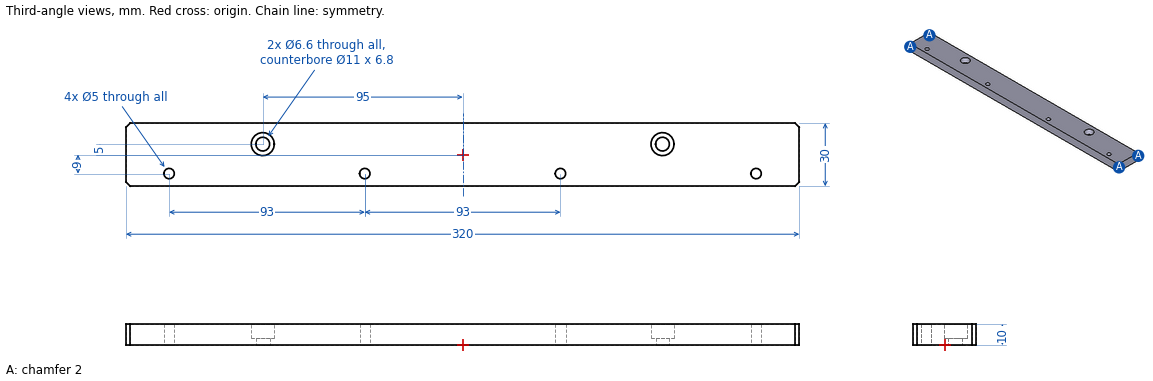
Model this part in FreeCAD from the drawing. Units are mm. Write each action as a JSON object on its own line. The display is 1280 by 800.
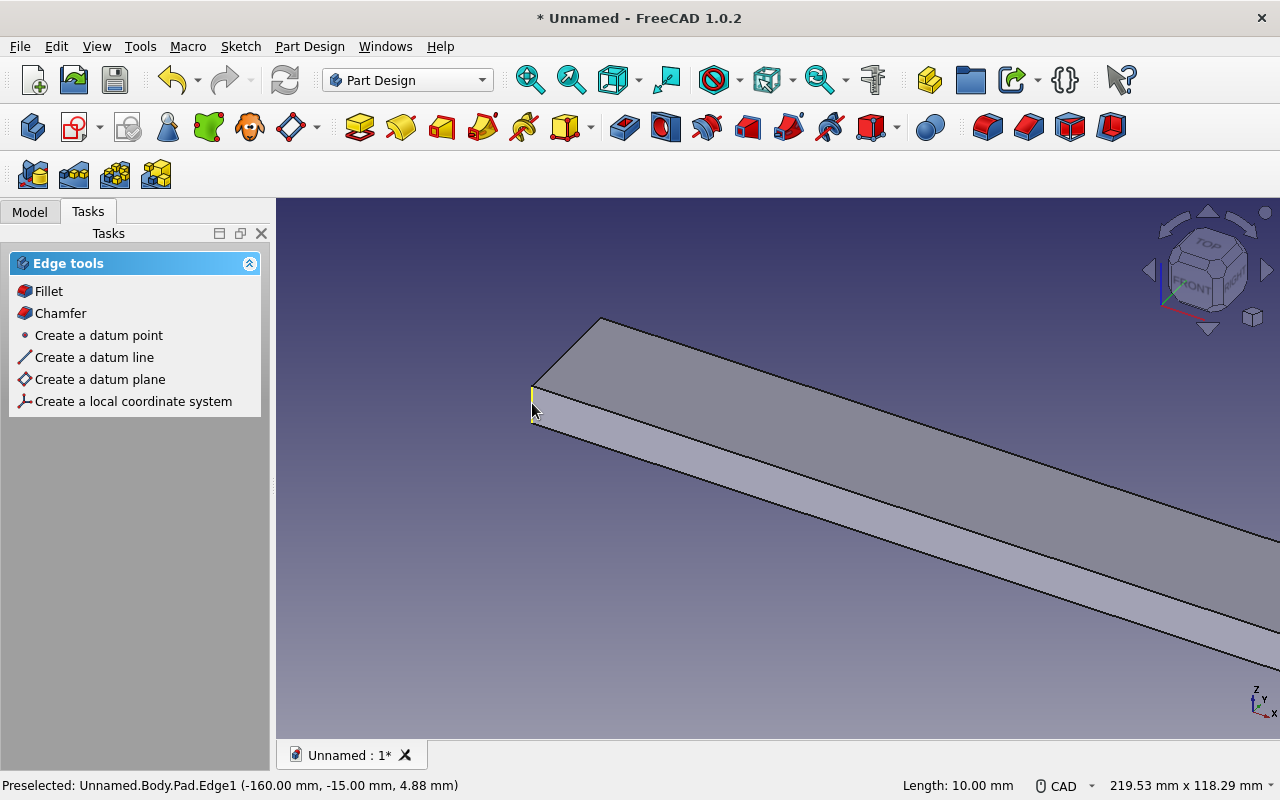
{"action": "left_click", "coordinate": [531, 80]}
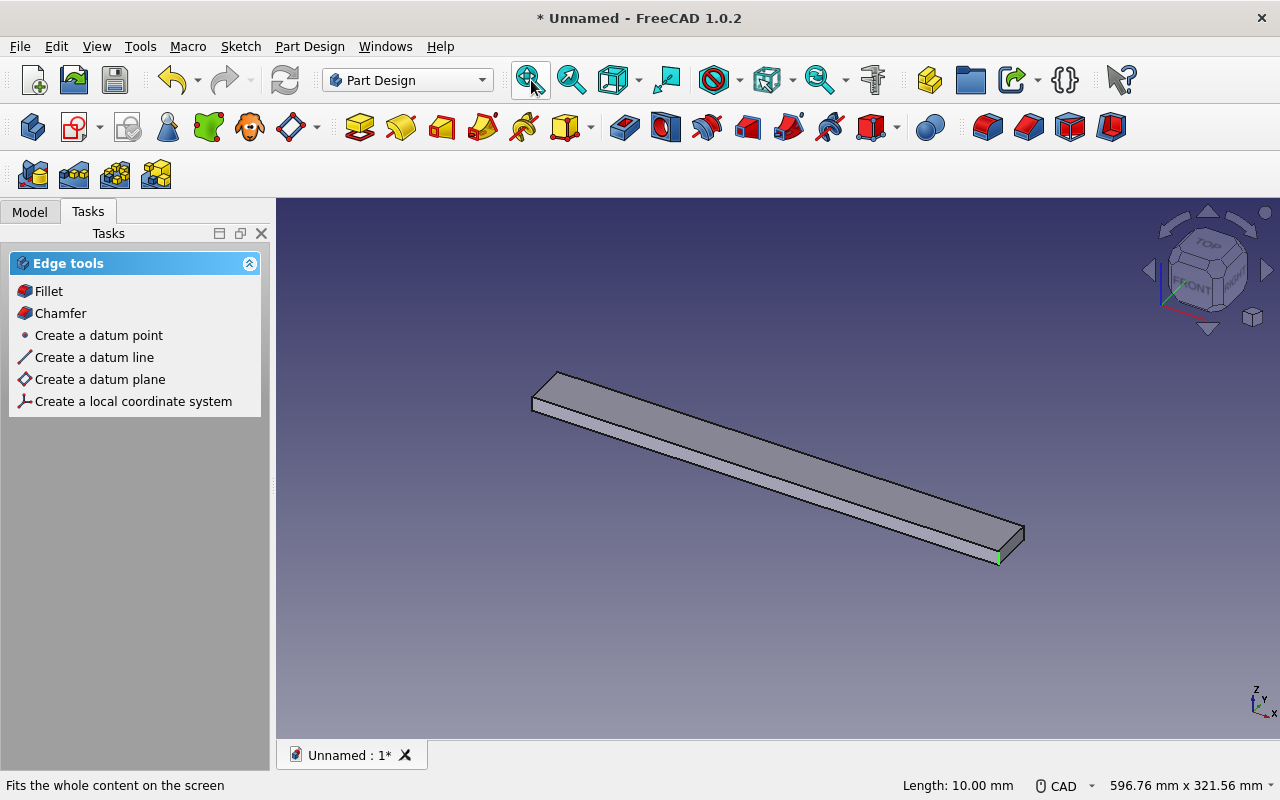
{"action": "key", "text": "0"}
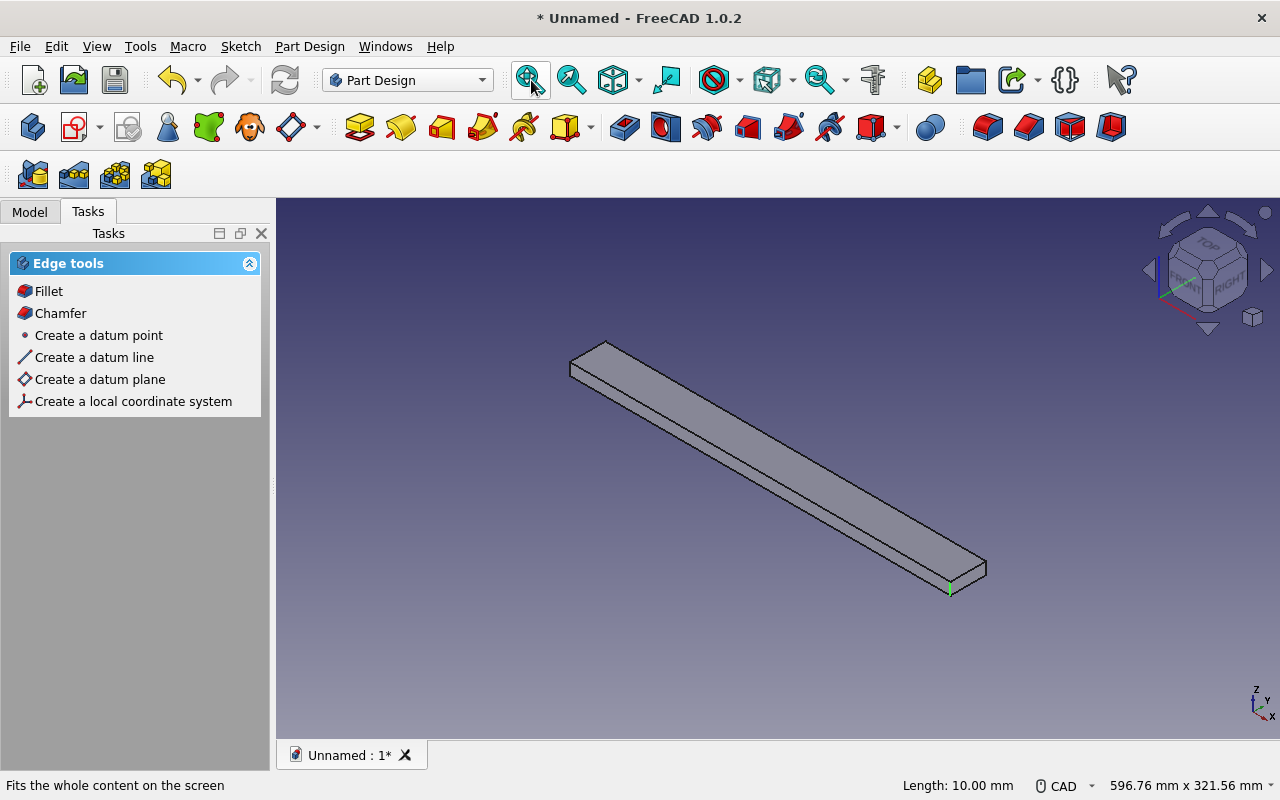
{"action": "scroll", "coordinate": [570, 368], "scroll_direction": "up", "scroll_amount": 5}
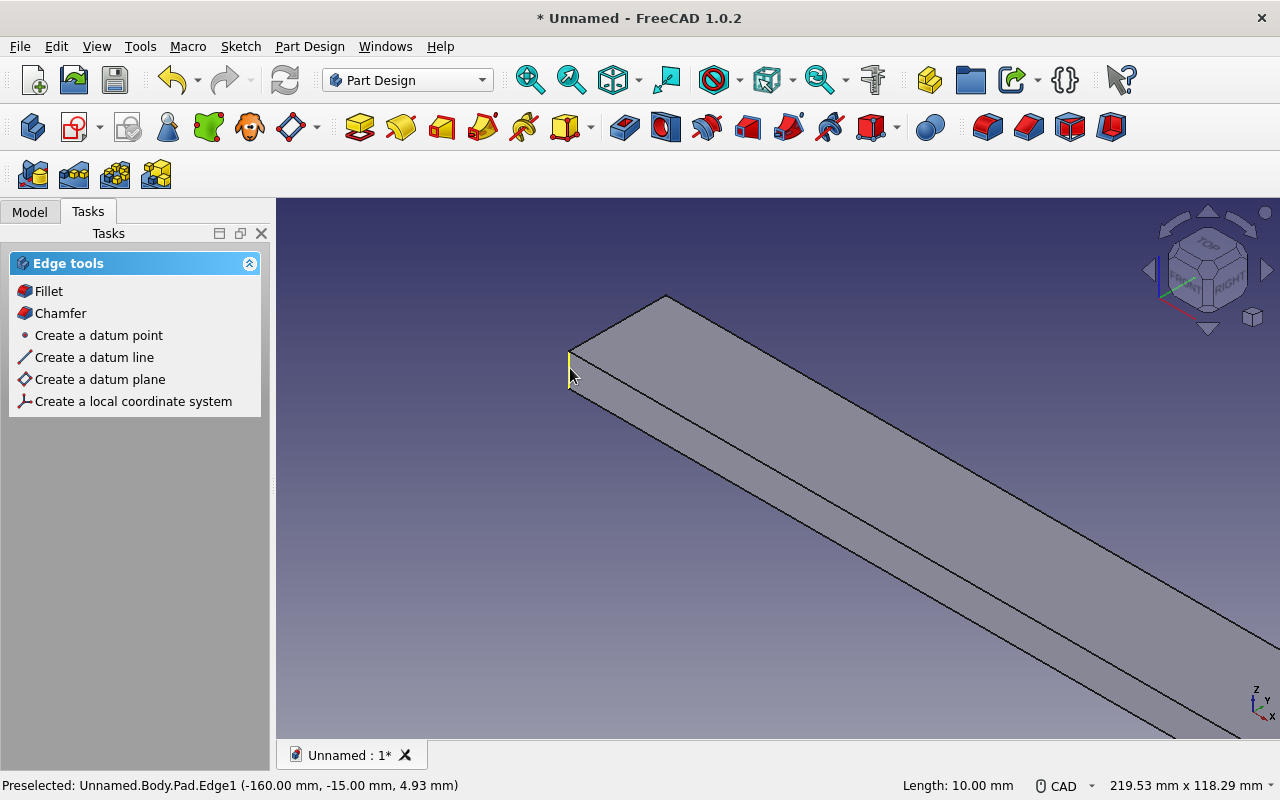
{"action": "left_click", "coordinate": [531, 80]}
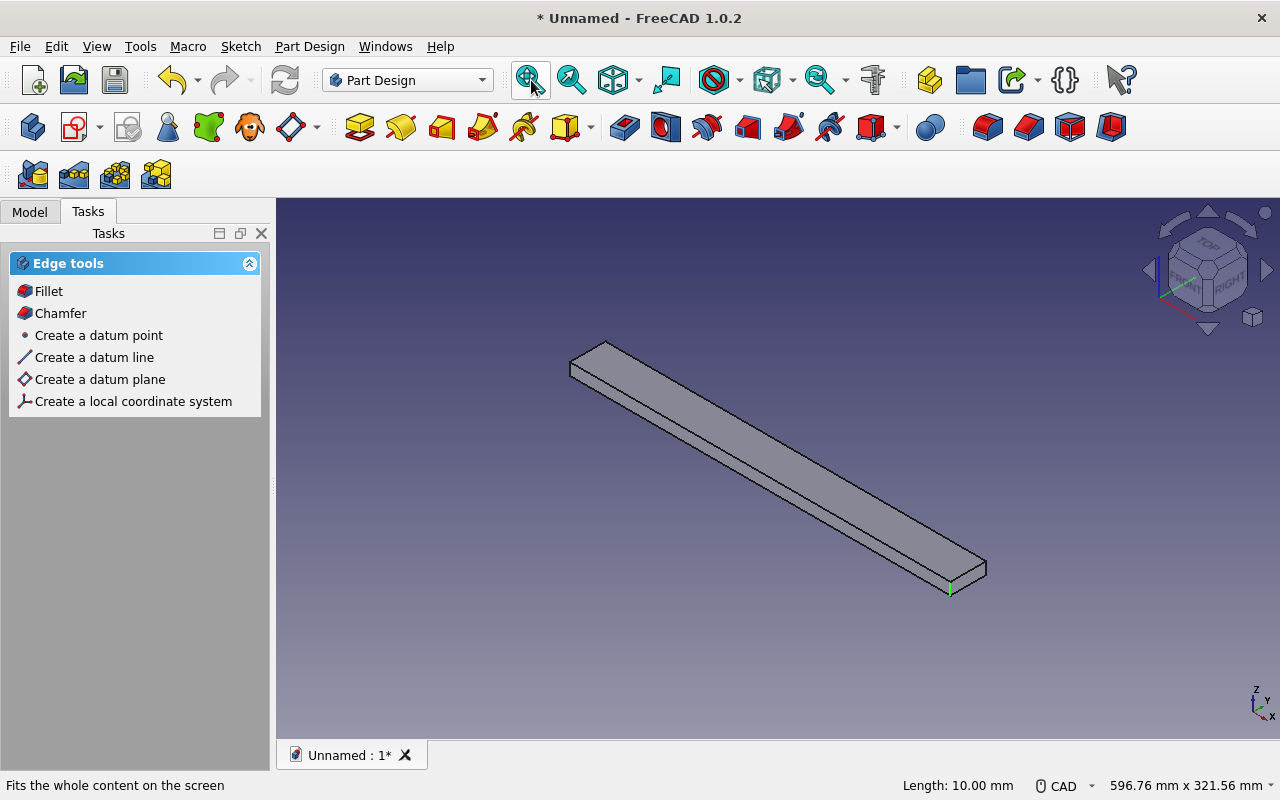
{"action": "key", "text": "2"}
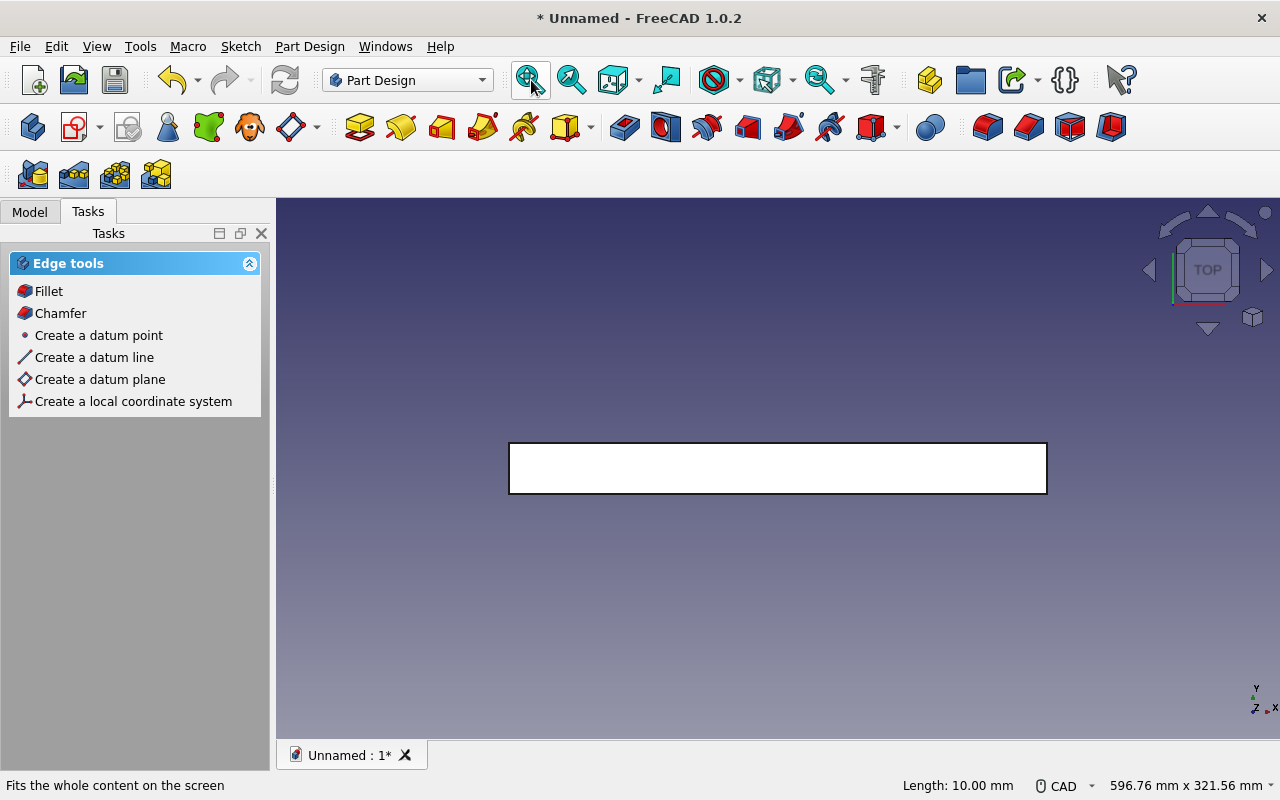
{"action": "scroll", "coordinate": [509, 493], "scroll_direction": "up", "scroll_amount": 5}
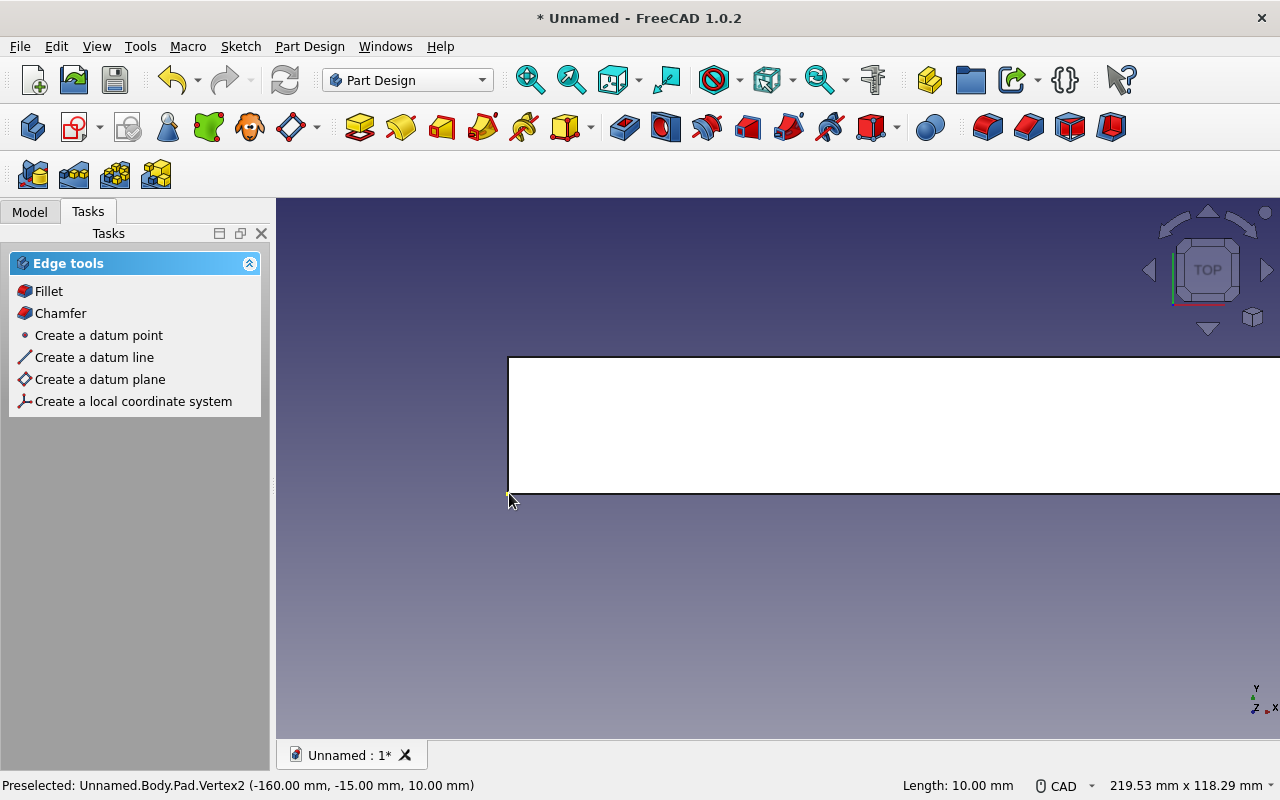
{"action": "left_click", "coordinate": [531, 80]}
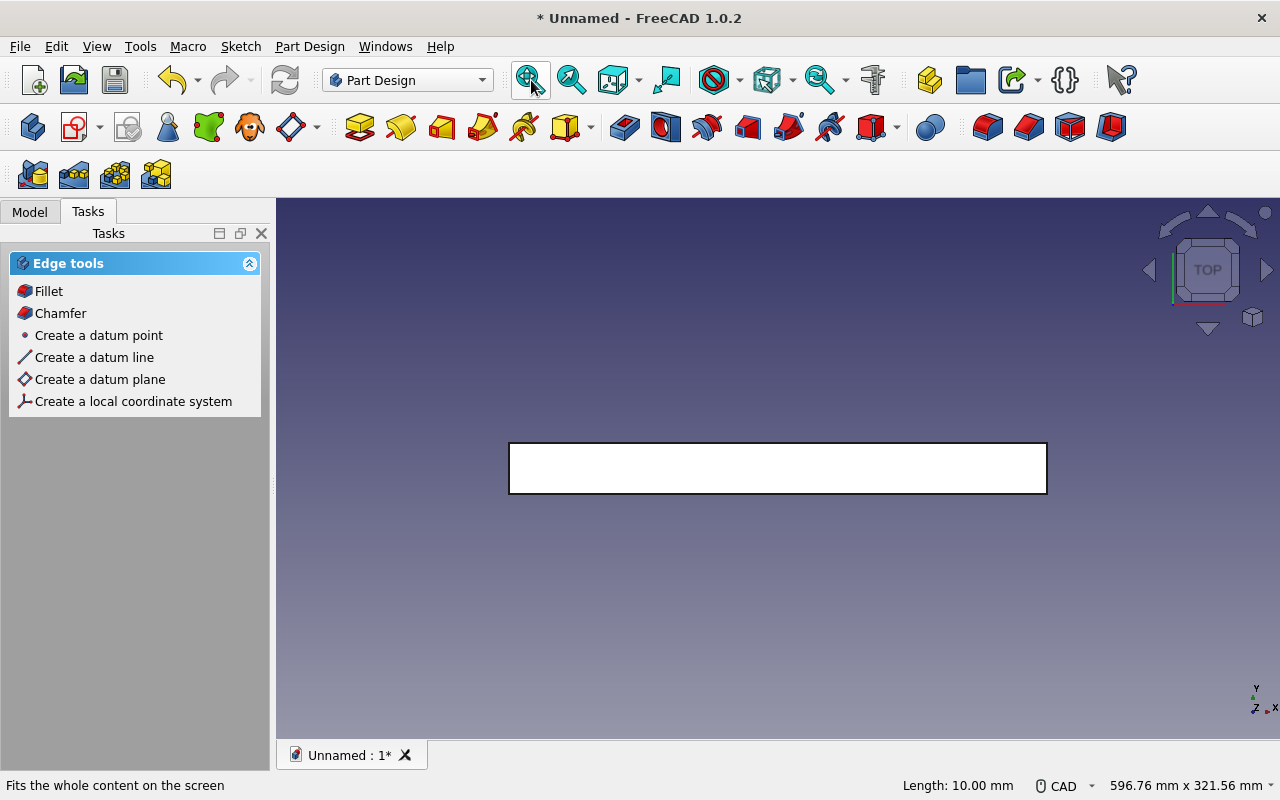
{"action": "key", "text": "1"}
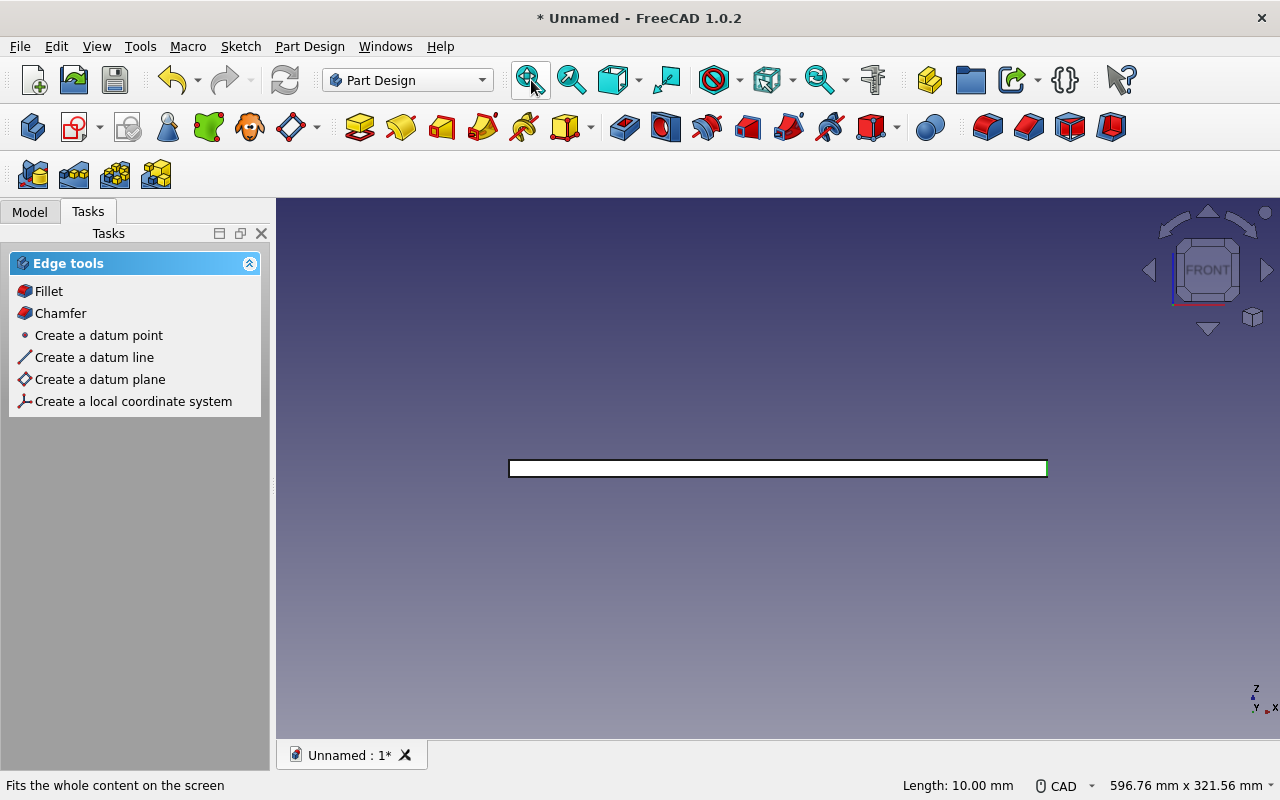
{"action": "left_click", "coordinate": [509, 467], "text": "ctrl"}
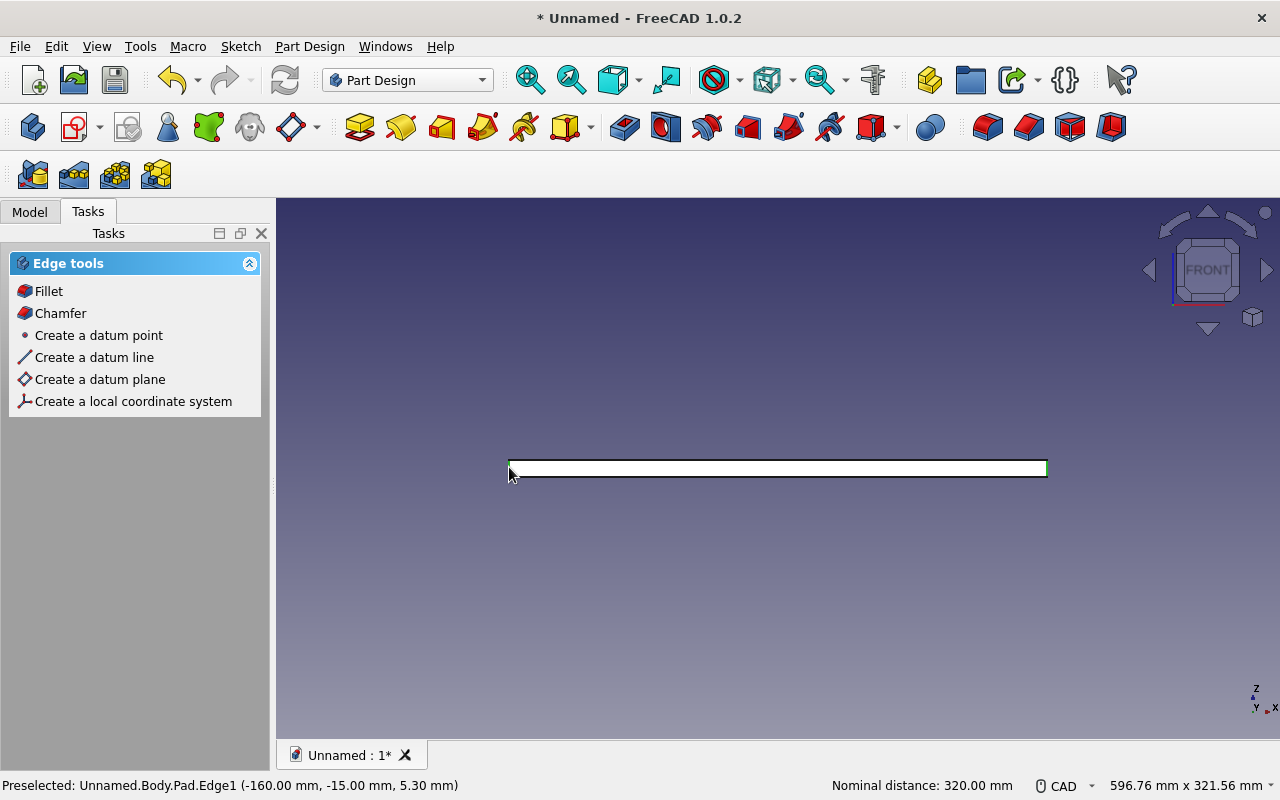
{"action": "scroll", "coordinate": [509, 467], "scroll_direction": "up", "scroll_amount": 5}